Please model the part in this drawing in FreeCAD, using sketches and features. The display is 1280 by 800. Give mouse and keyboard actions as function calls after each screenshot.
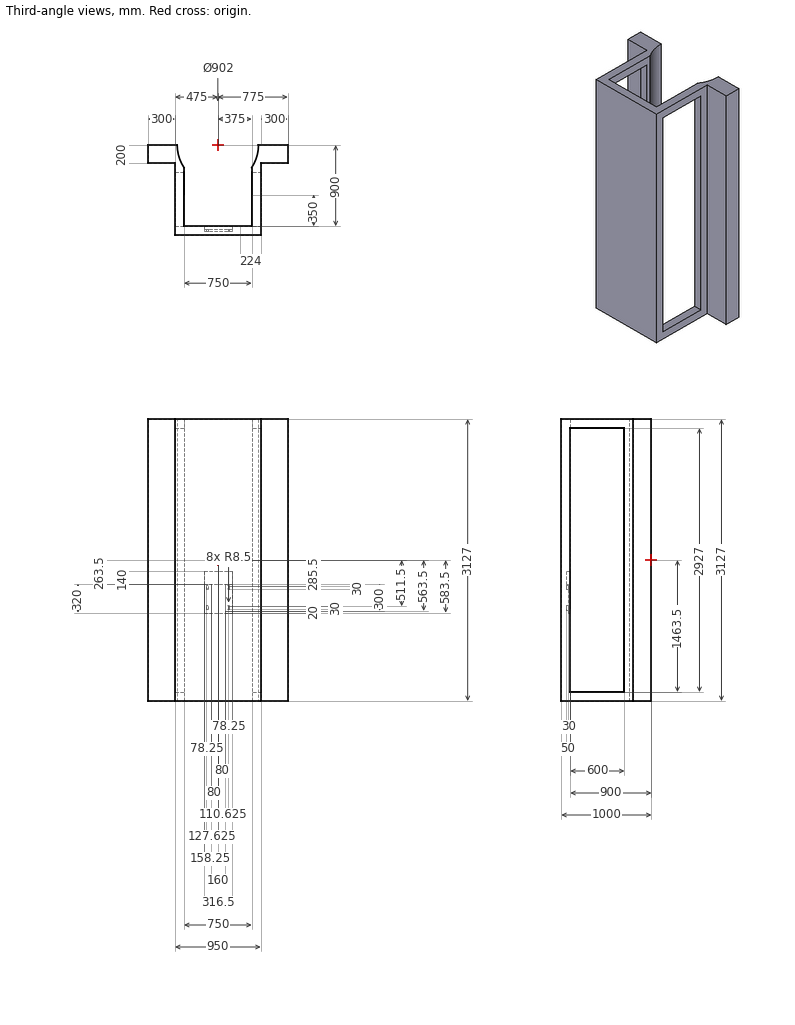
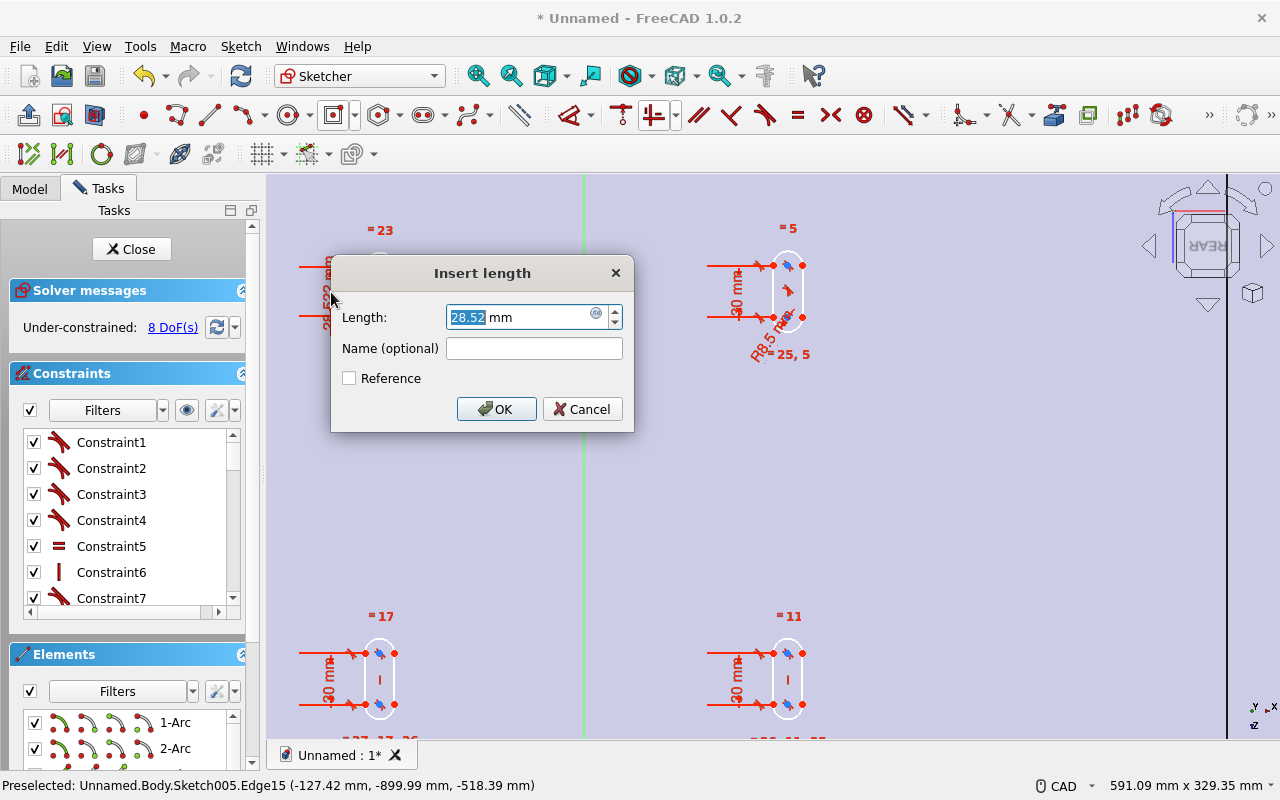
text(30)
key(Return)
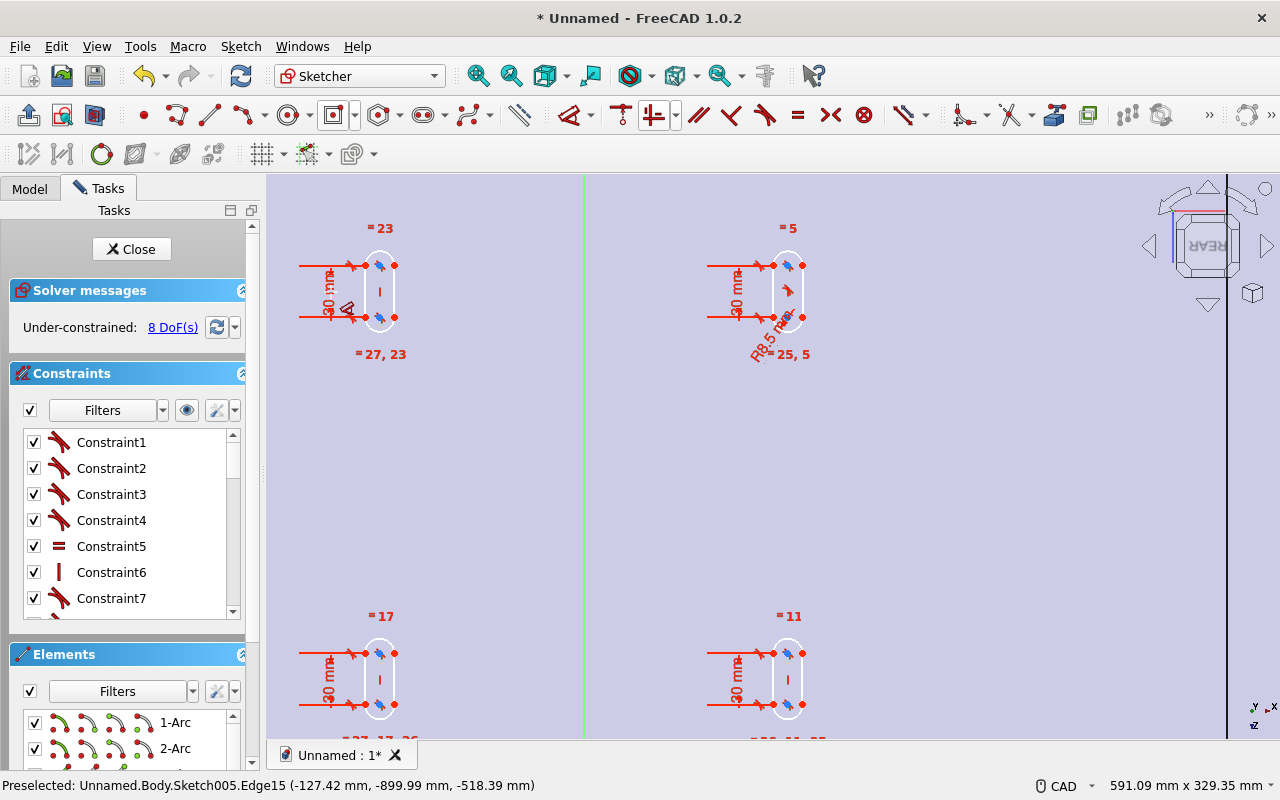
click(773, 317)
click(807, 514)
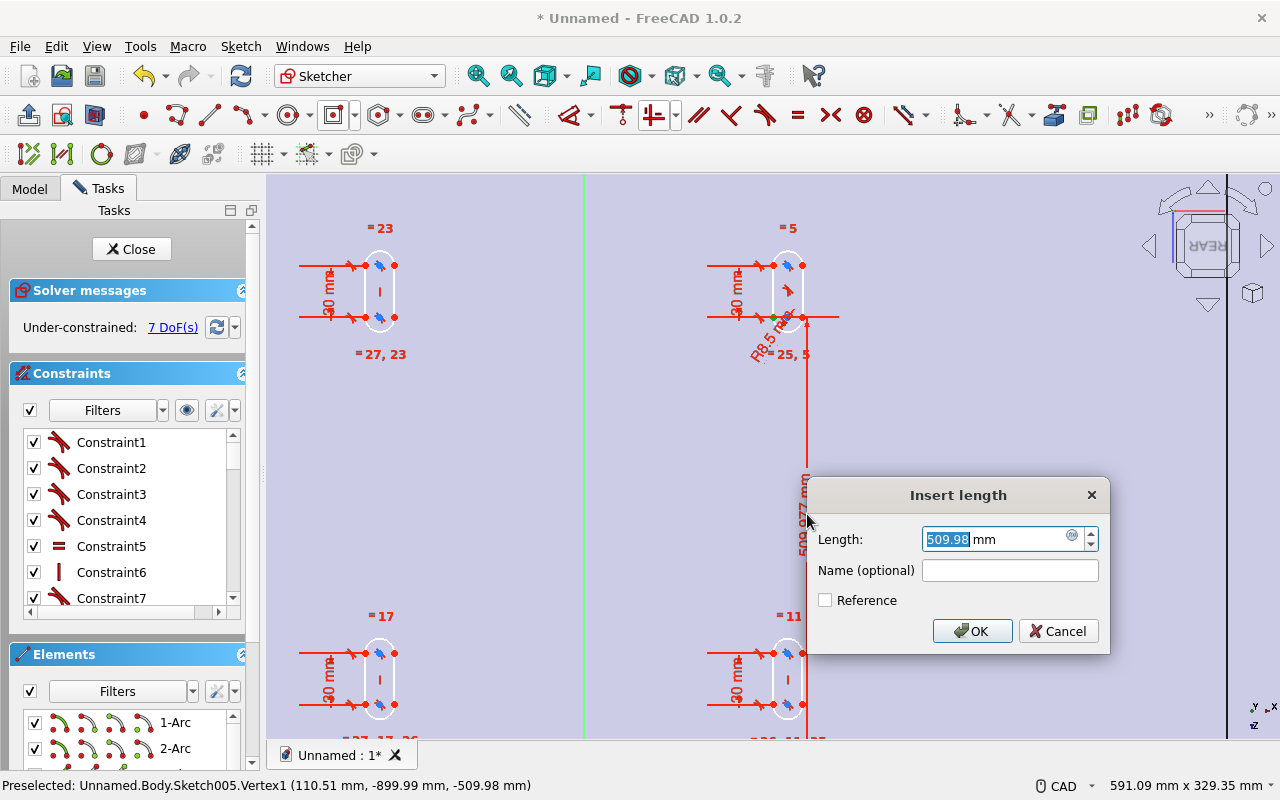
text(511.5)
key(Return)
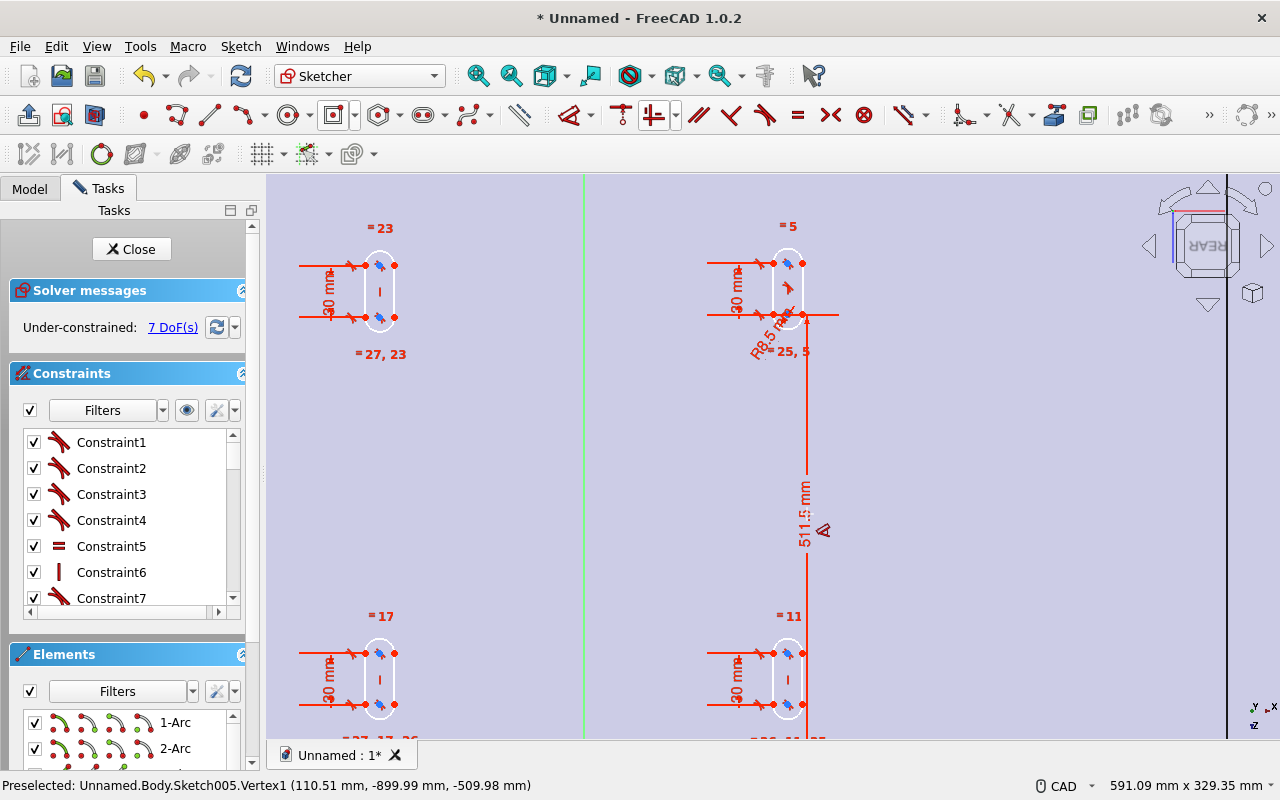
click(773, 705)
click(550, 708)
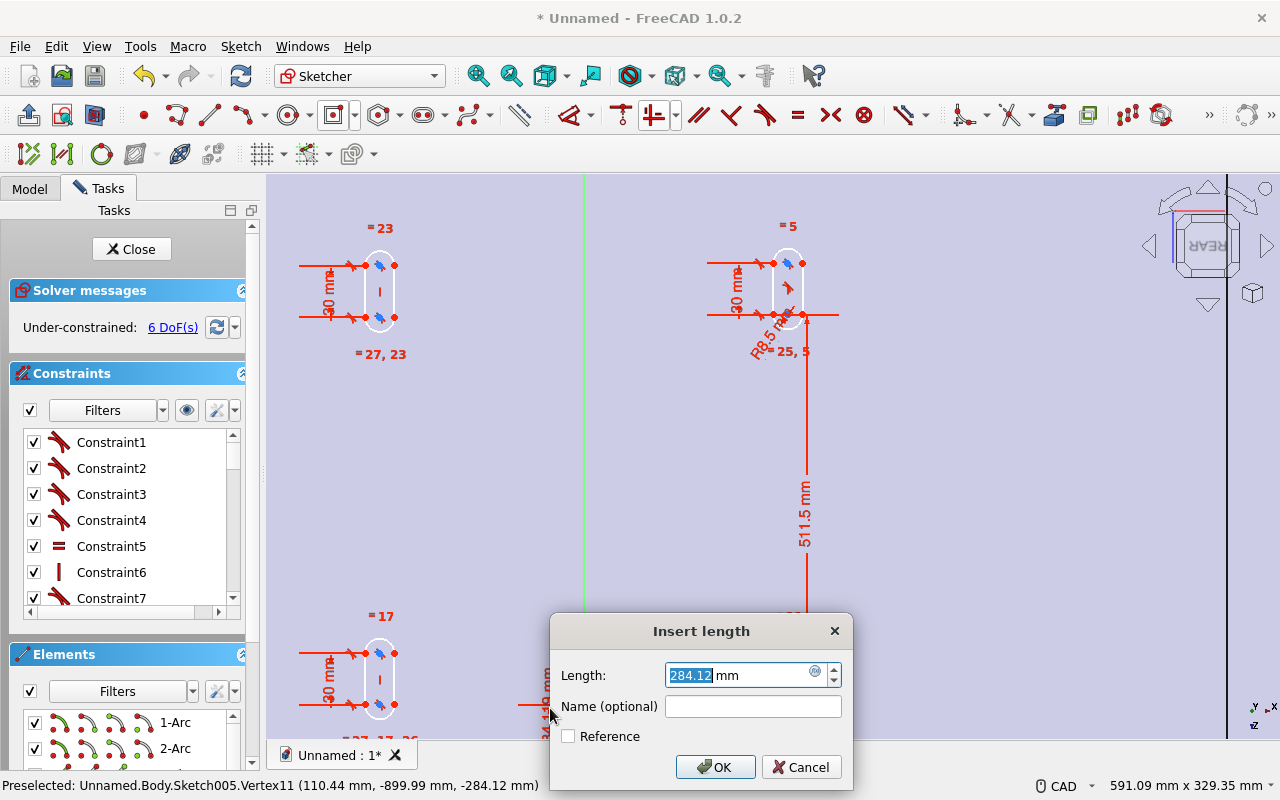
text(285.5)
key(Return)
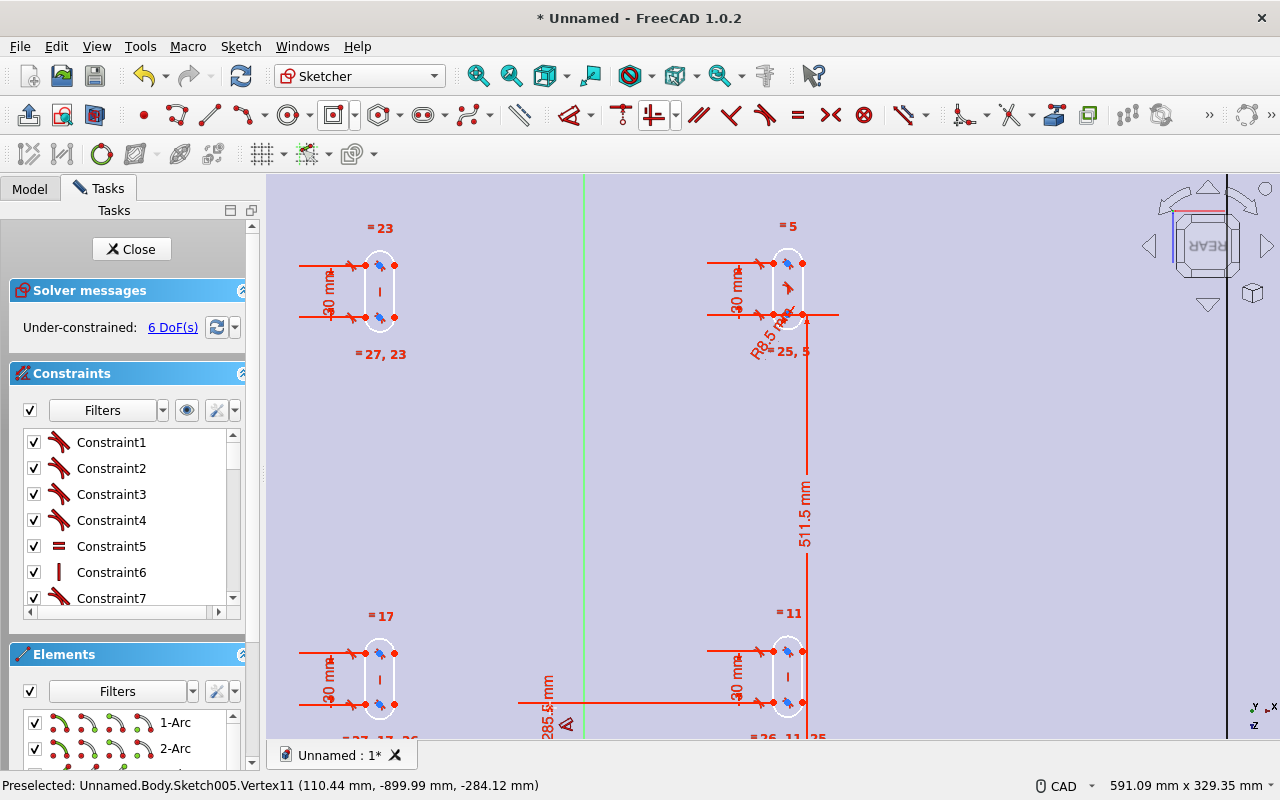
click(365, 705)
click(331, 708)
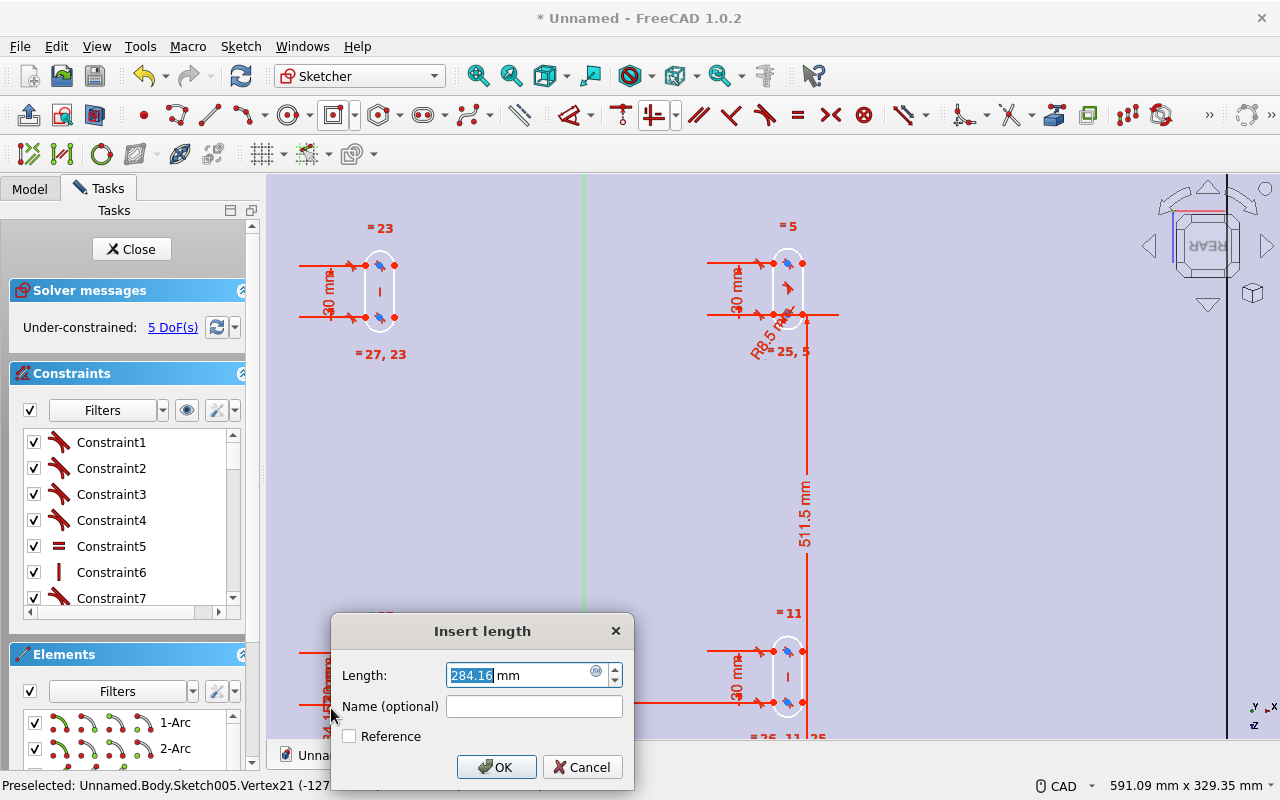
text(285.5)
key(Return)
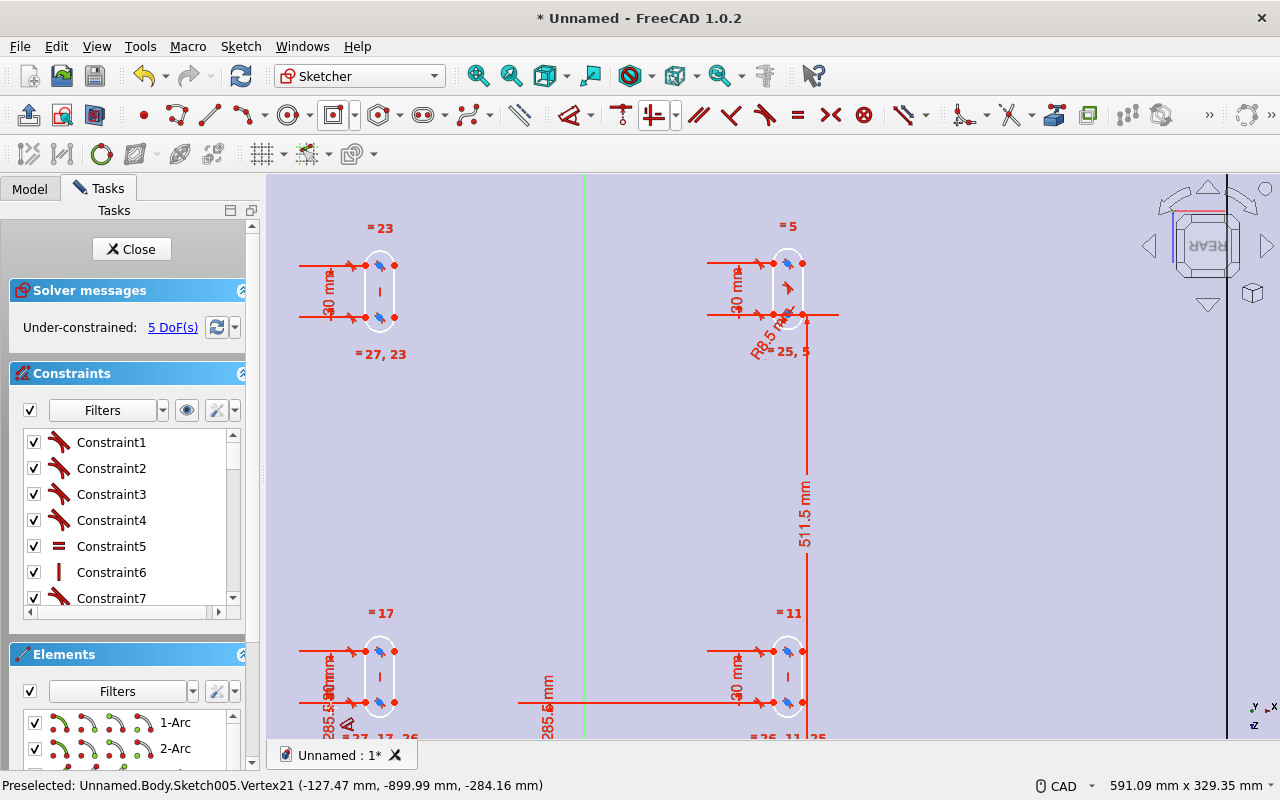
click(365, 317)
click(331, 514)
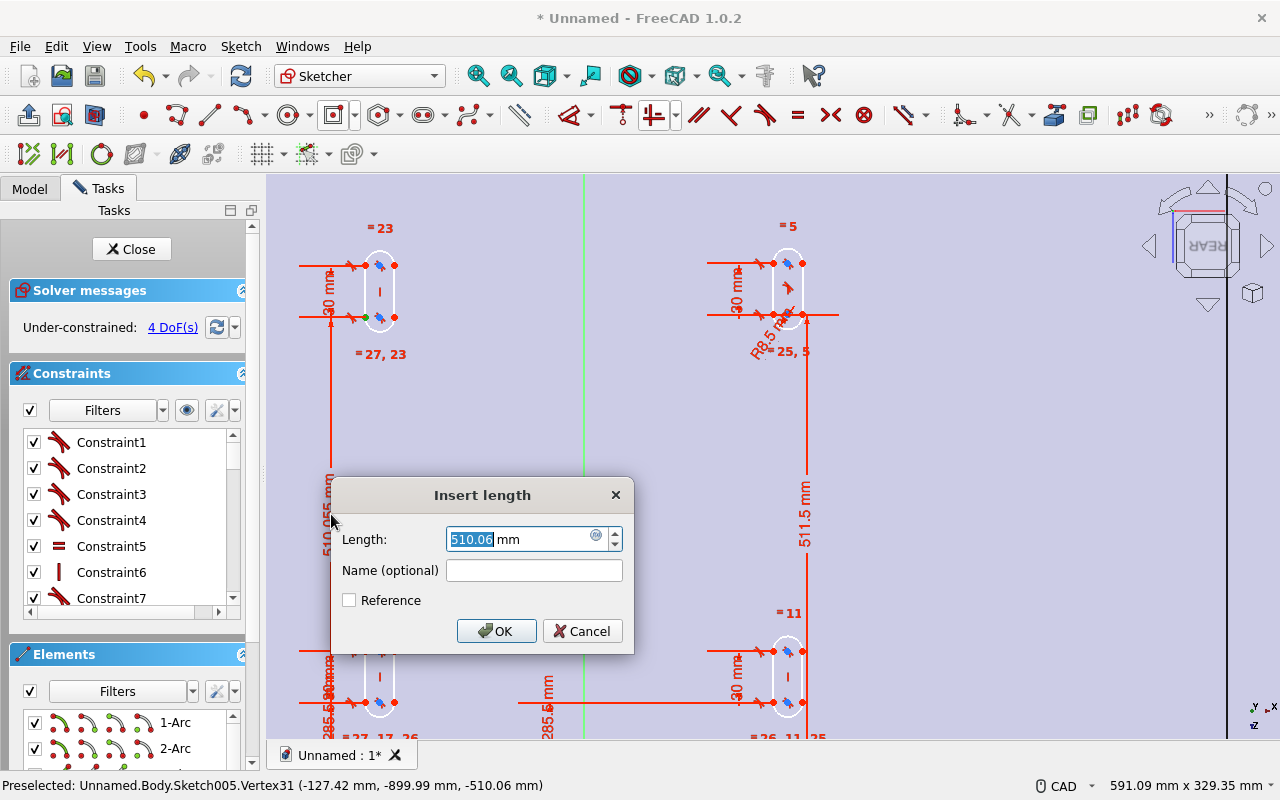
text(511.5)
key(Return)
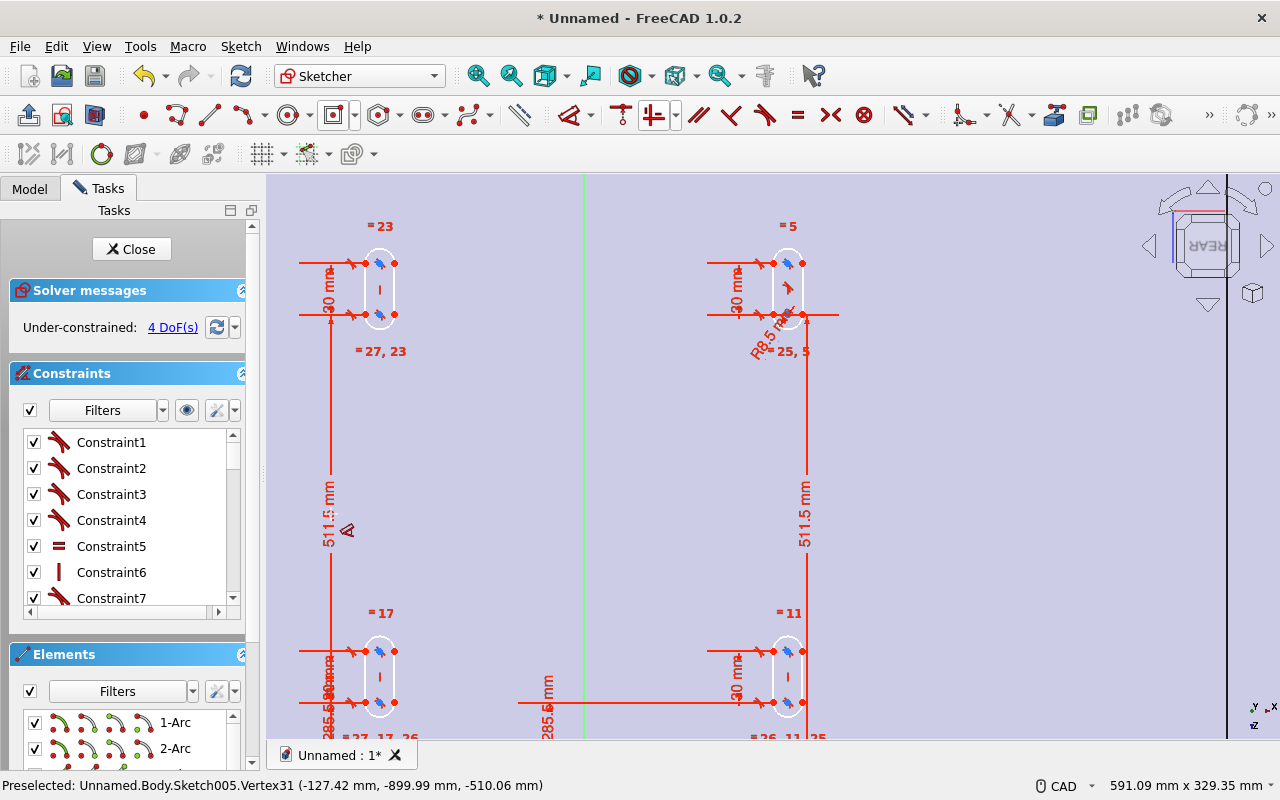
click(773, 315)
click(635, 281)